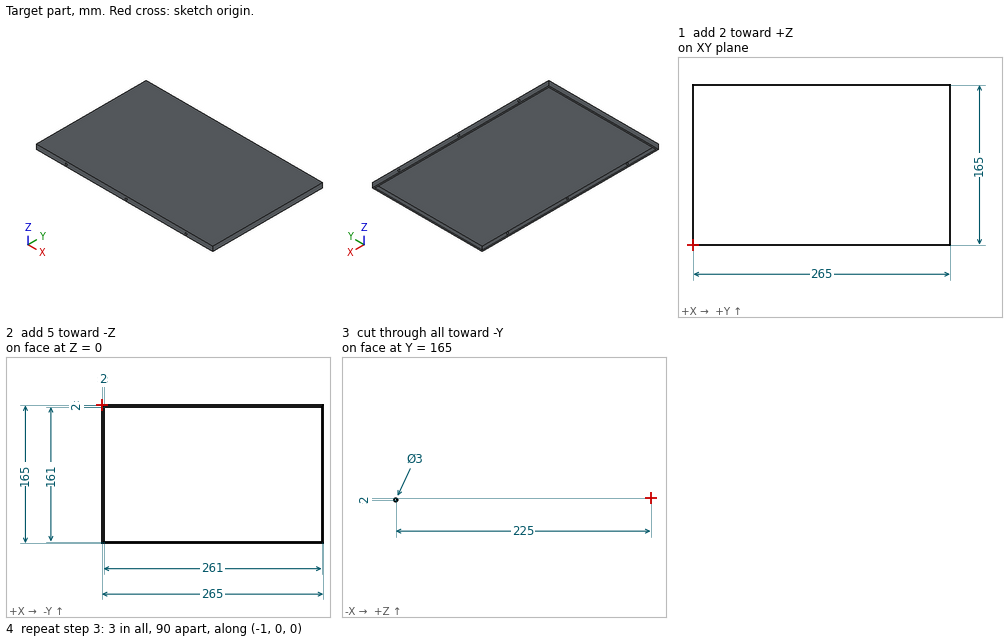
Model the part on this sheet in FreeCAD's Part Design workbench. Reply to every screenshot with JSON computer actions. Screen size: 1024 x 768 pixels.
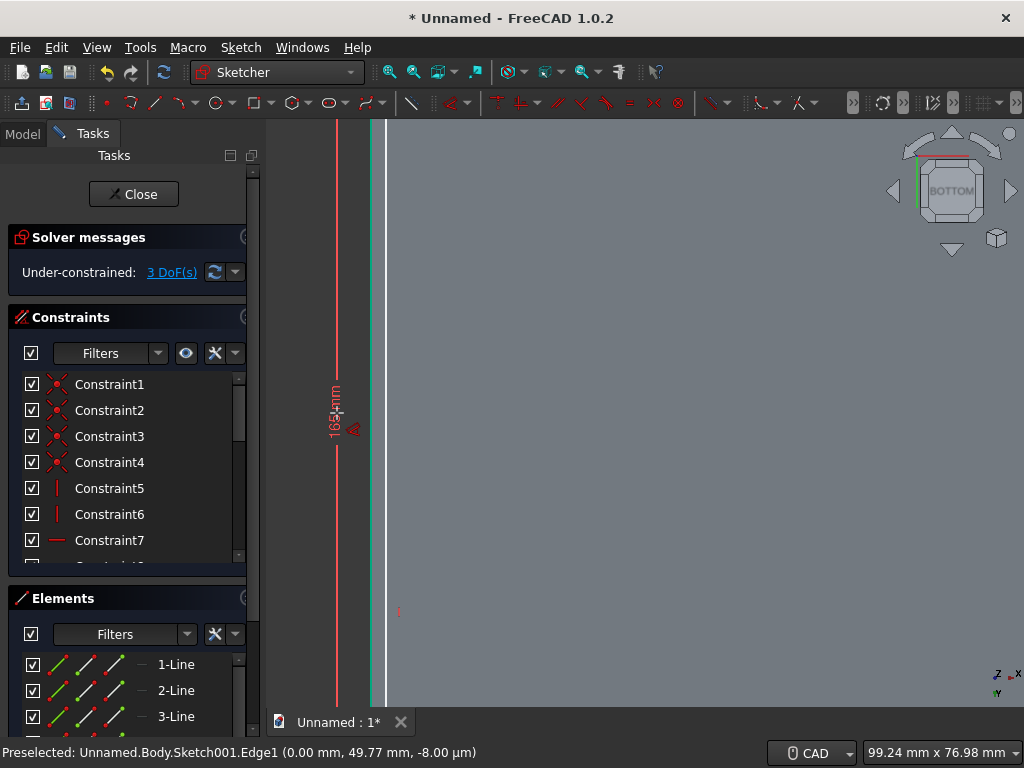
{"action": "scroll", "coordinate": [372, 362], "scroll_direction": "down", "scroll_amount": 8}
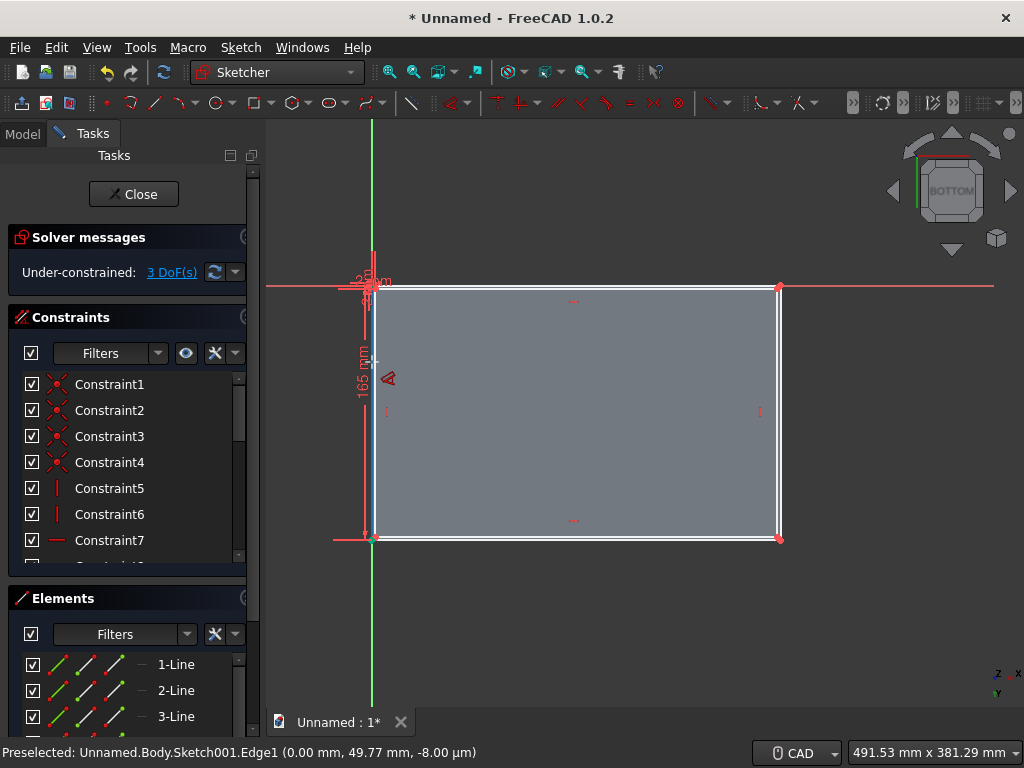
{"action": "scroll", "coordinate": [495, 540], "scroll_direction": "up", "scroll_amount": 8}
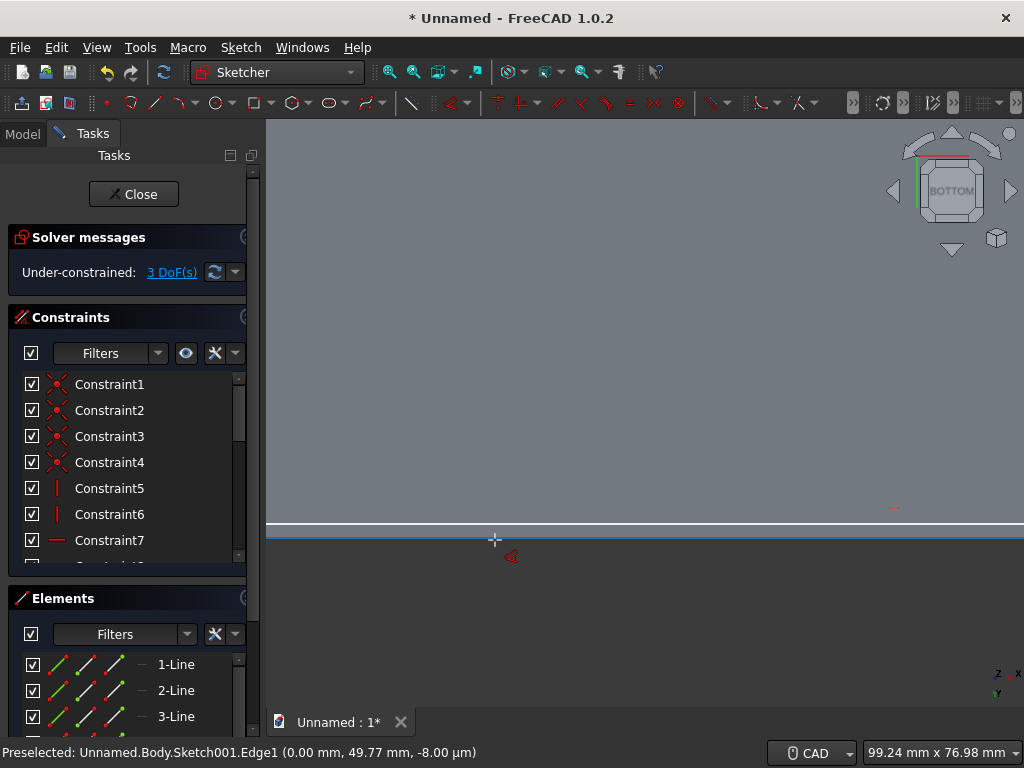
{"action": "left_click", "coordinate": [492, 538]}
{"action": "left_click", "coordinate": [576, 572]}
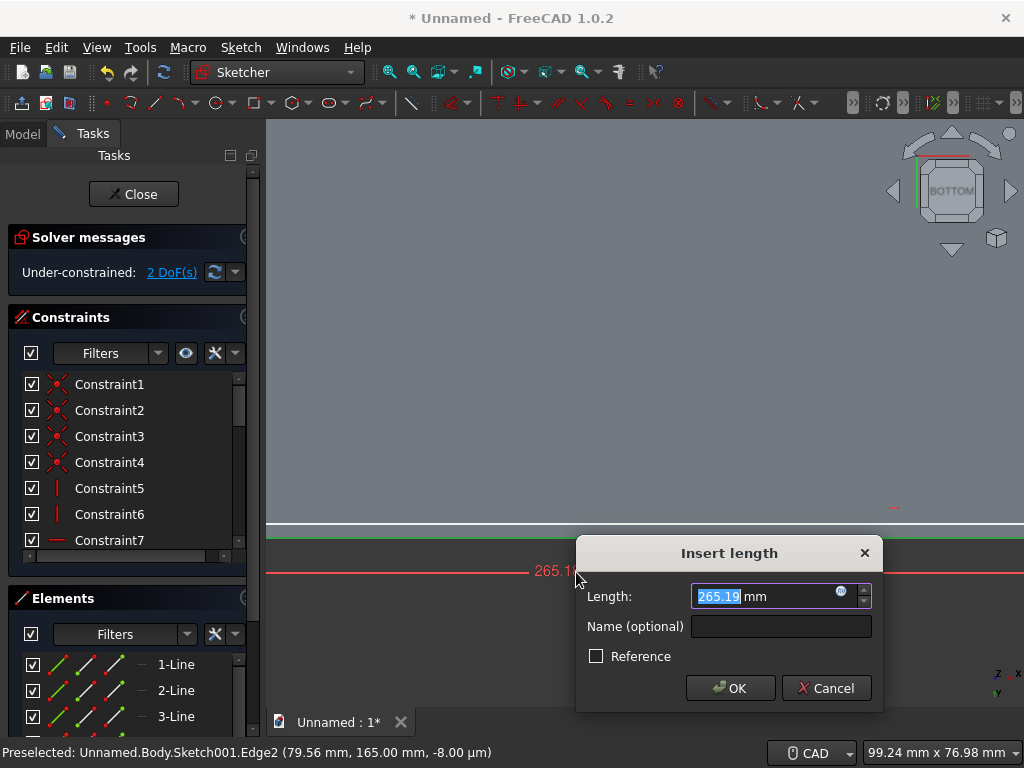
{"action": "type", "text": "265"}
{"action": "key", "text": "Return"}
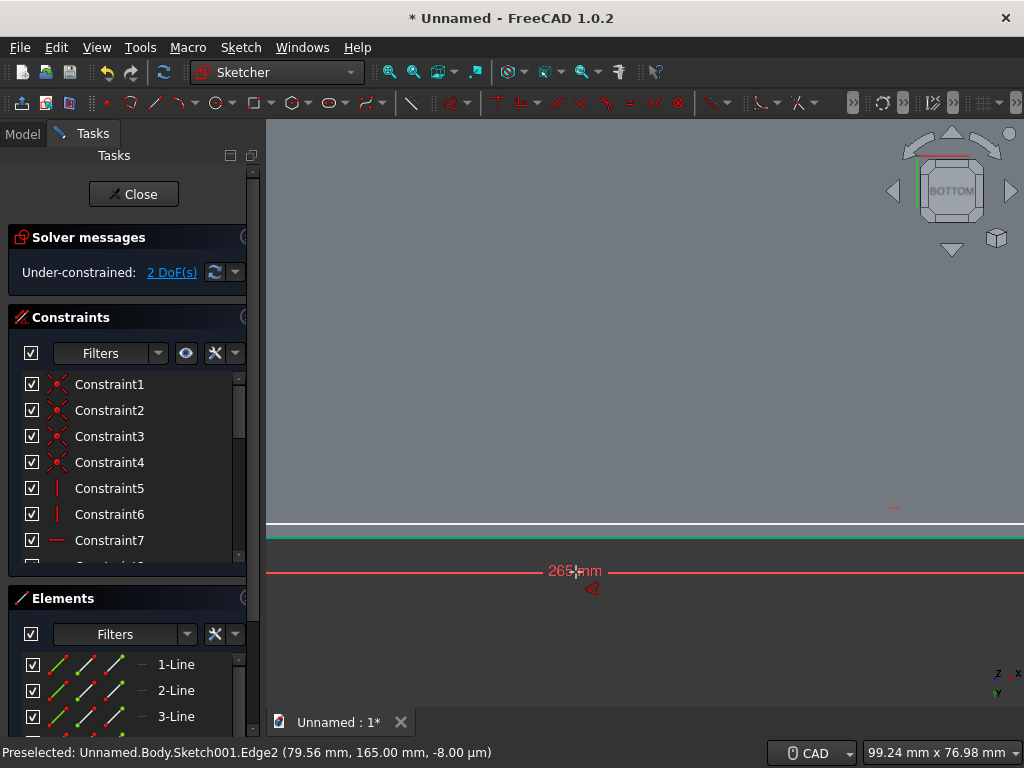
{"action": "scroll", "coordinate": [496, 541], "scroll_direction": "down", "scroll_amount": 8}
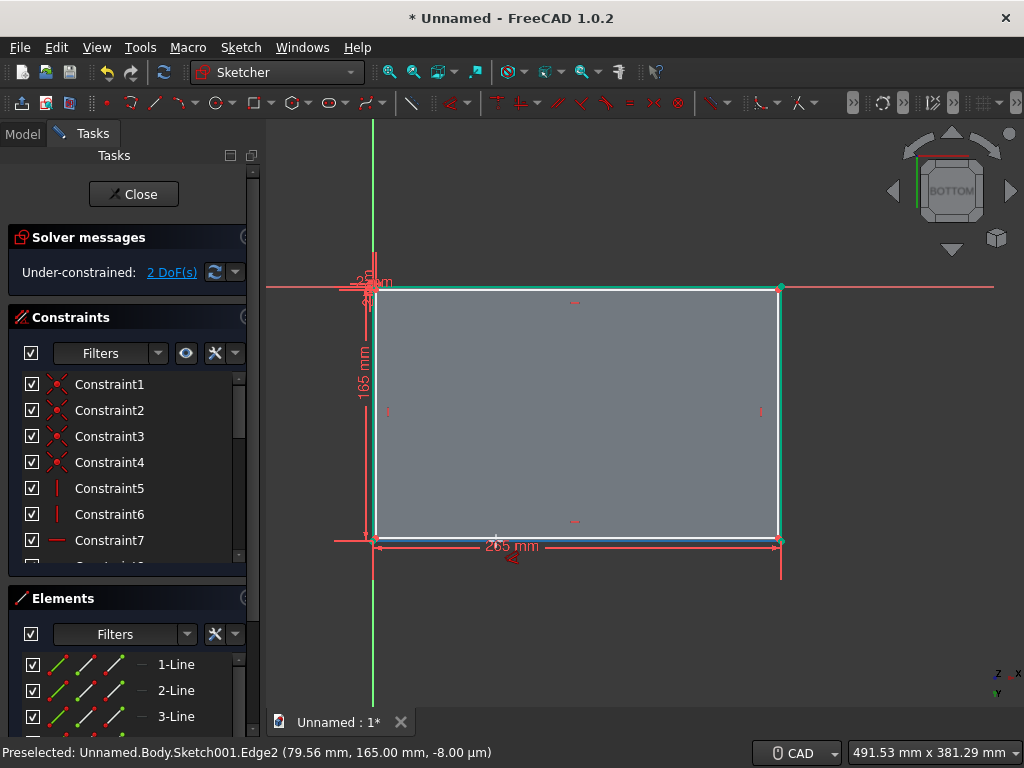
{"action": "scroll", "coordinate": [376, 364], "scroll_direction": "up", "scroll_amount": 8}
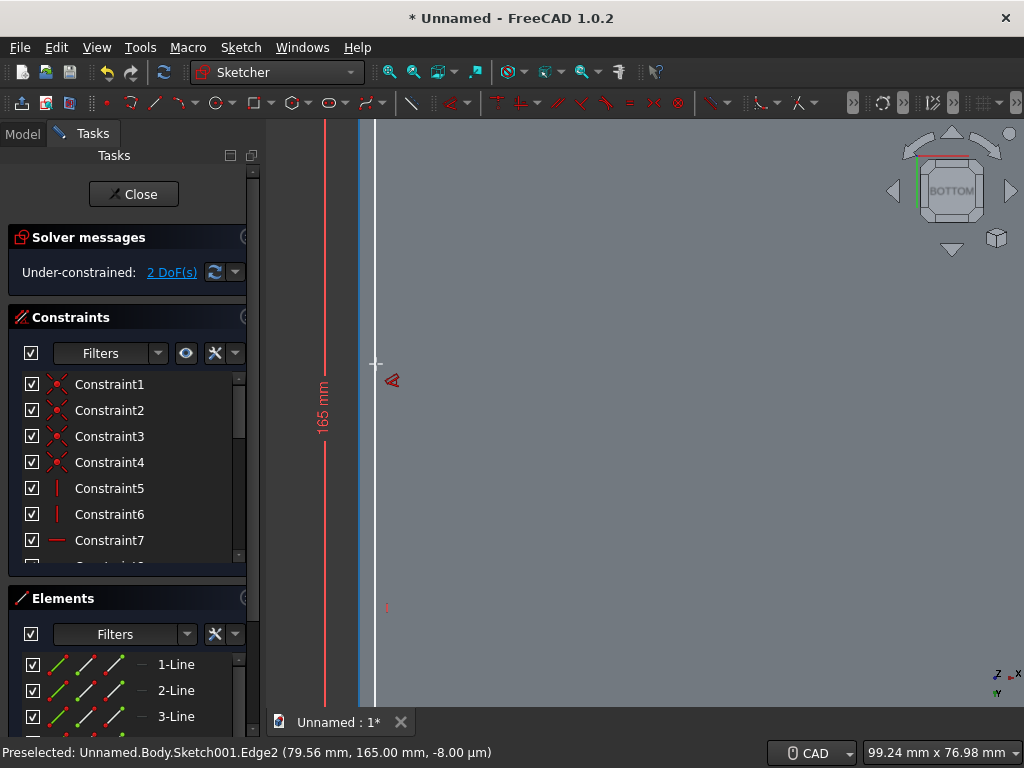
{"action": "left_click", "coordinate": [375, 363]}
{"action": "left_click", "coordinate": [341, 291]}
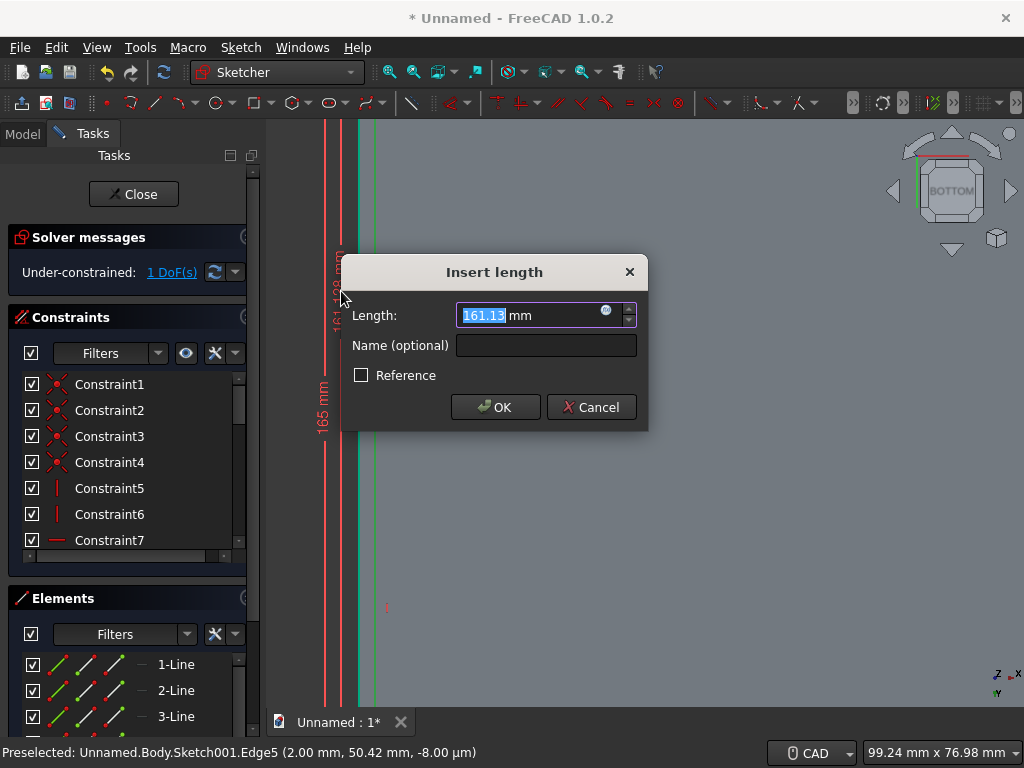
{"action": "type", "text": "161"}
{"action": "key", "text": "Return"}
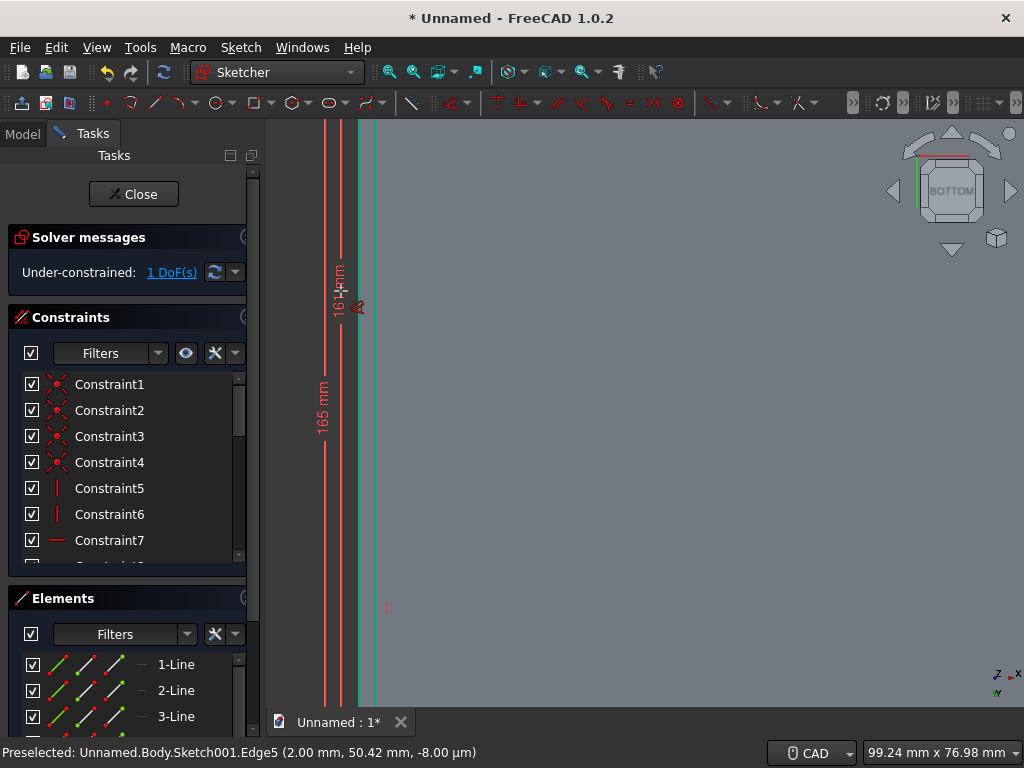
{"action": "scroll", "coordinate": [375, 363], "scroll_direction": "down", "scroll_amount": 8}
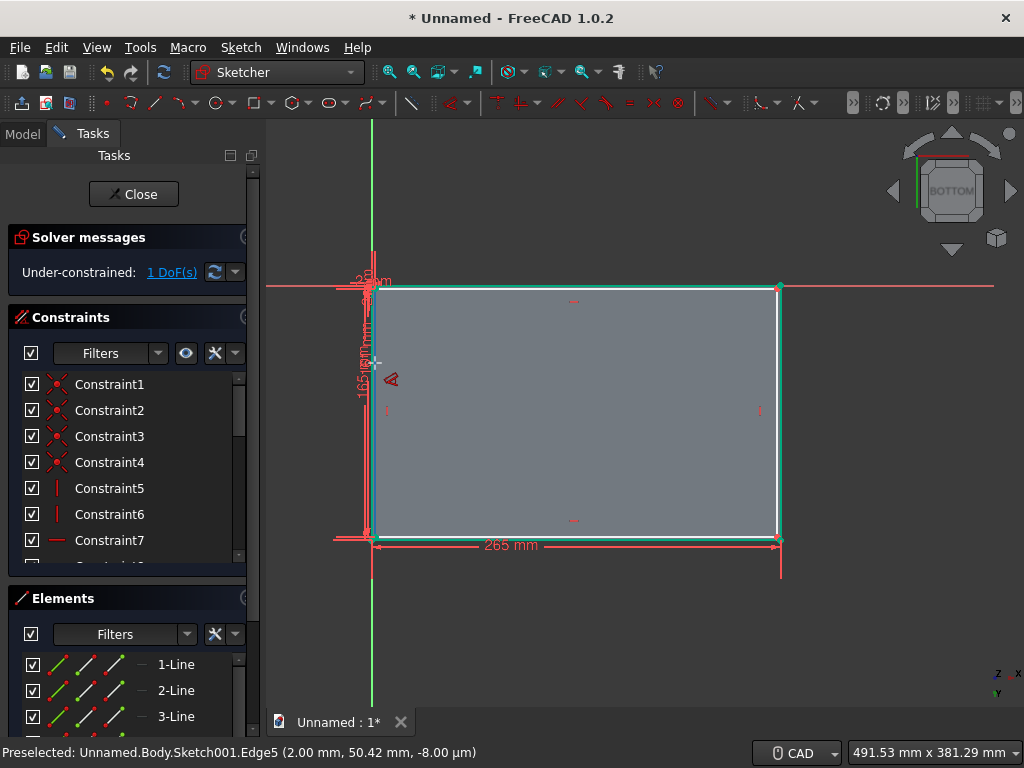
{"action": "scroll", "coordinate": [496, 537], "scroll_direction": "up", "scroll_amount": 8}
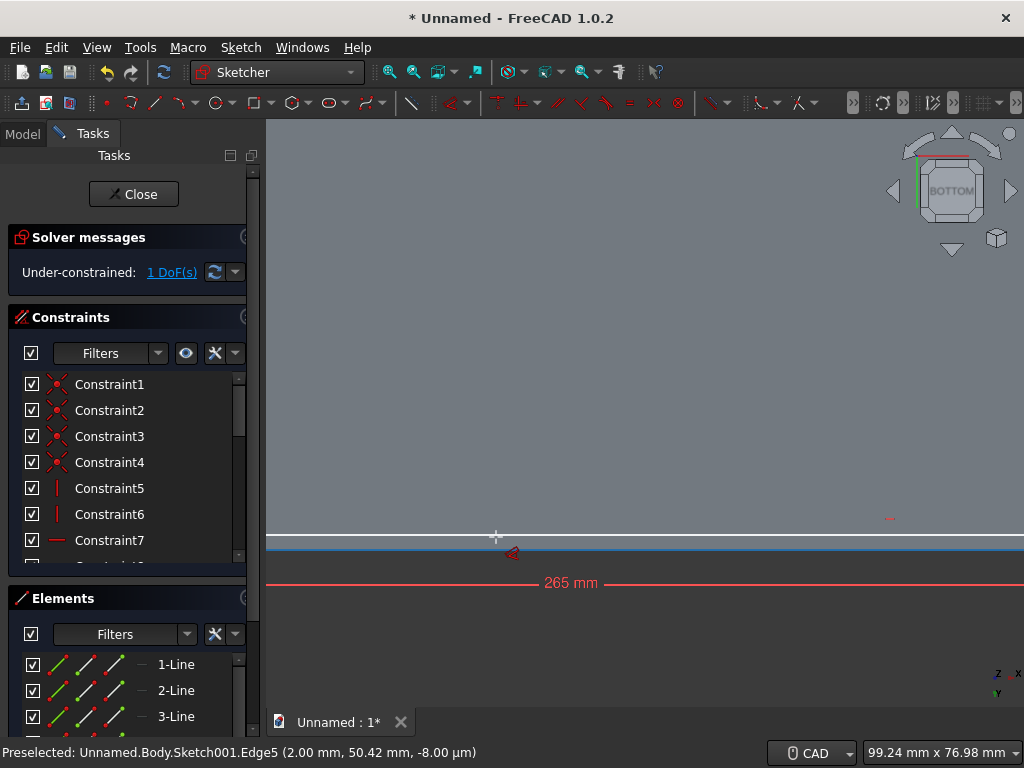
{"action": "left_click", "coordinate": [494, 535]}
{"action": "left_click", "coordinate": [447, 569]}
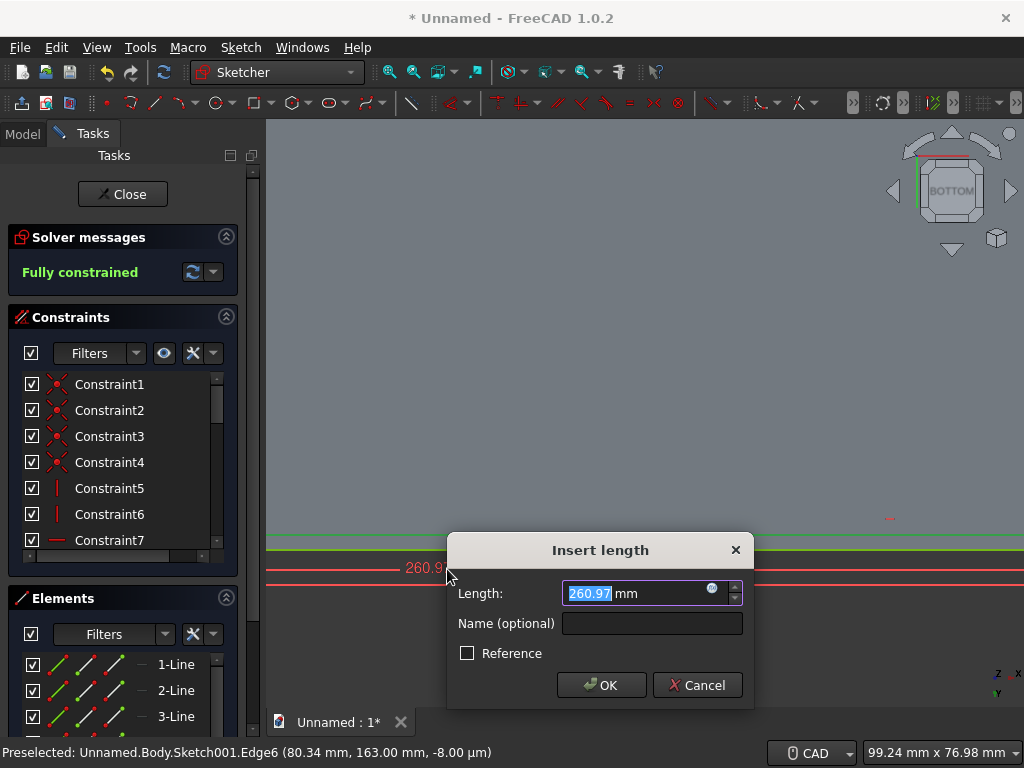
{"action": "type", "text": "261"}
{"action": "key", "text": "Return"}
{"action": "key", "text": "Escape"}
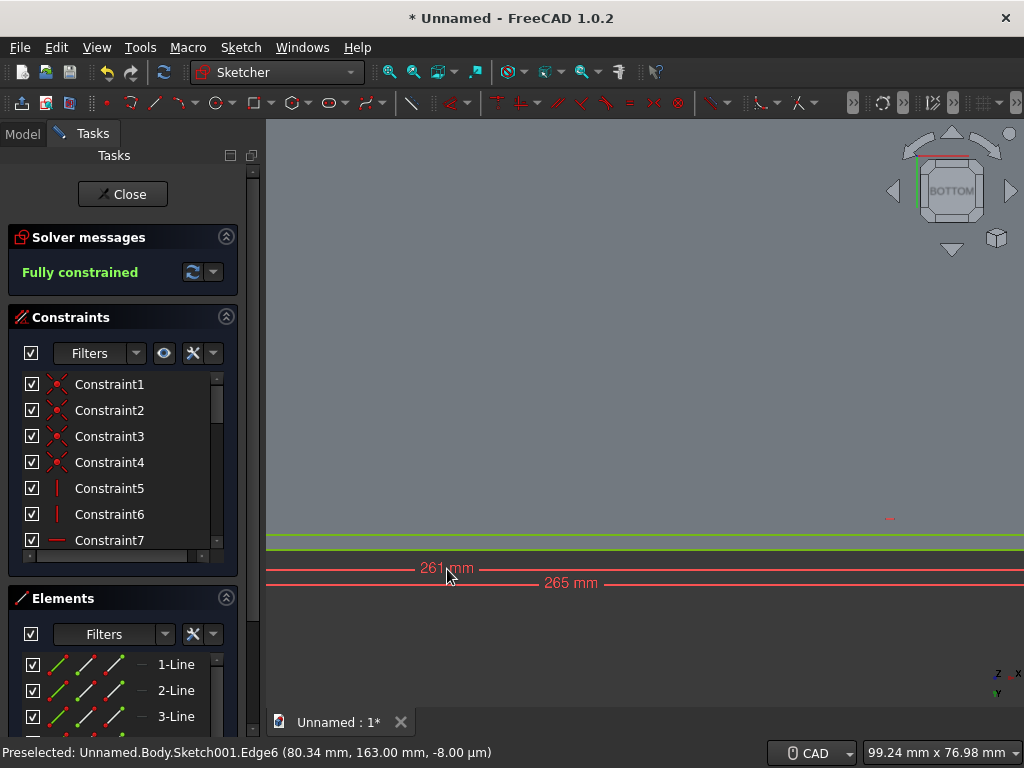
{"action": "left_click", "coordinate": [123, 194]}